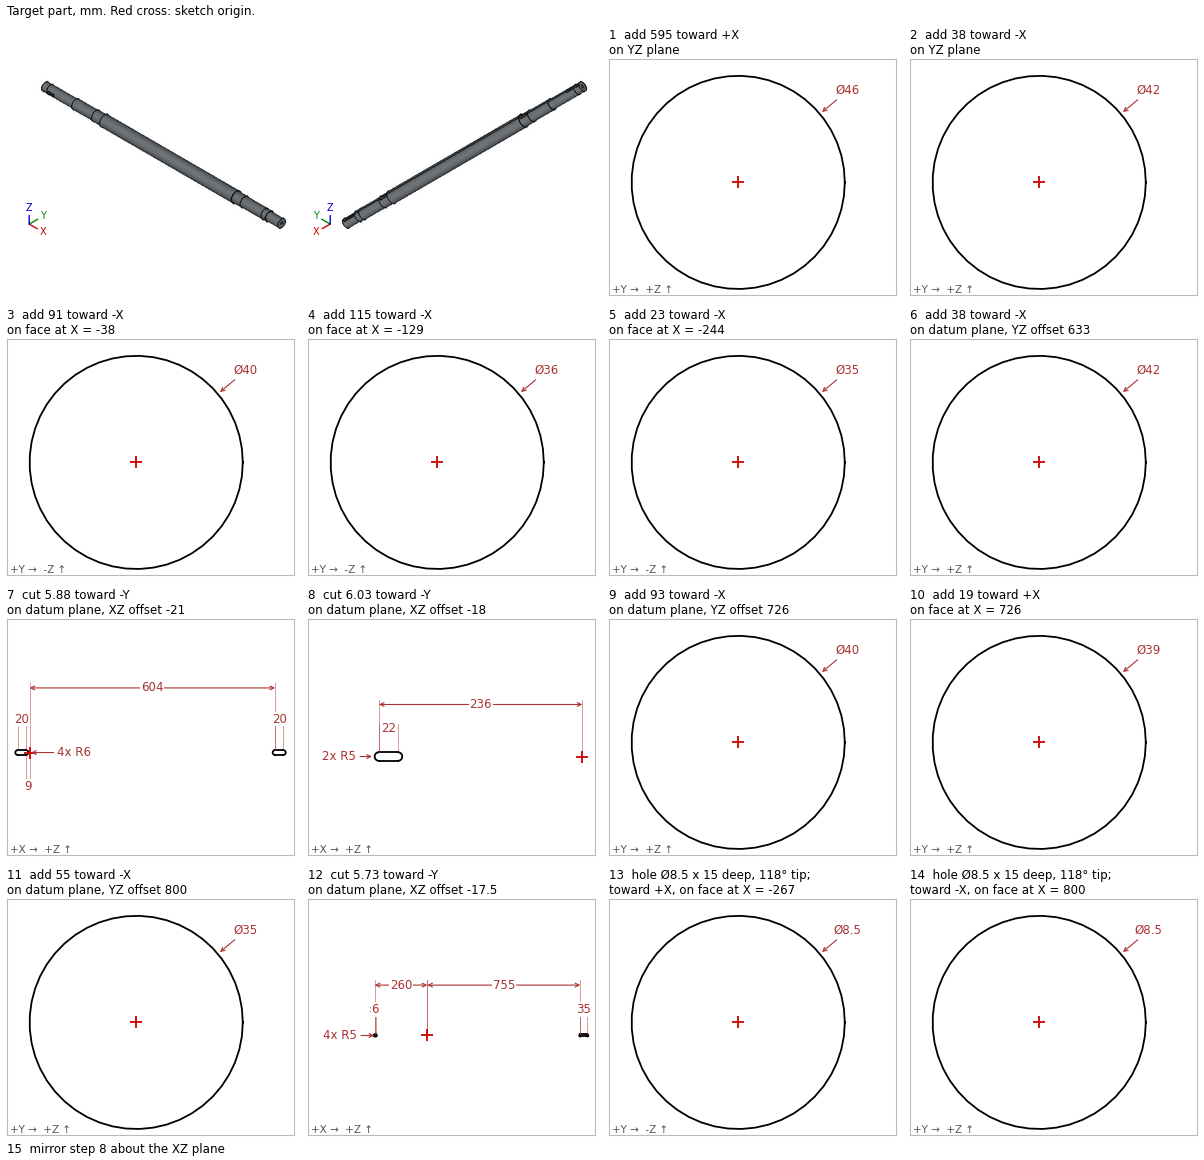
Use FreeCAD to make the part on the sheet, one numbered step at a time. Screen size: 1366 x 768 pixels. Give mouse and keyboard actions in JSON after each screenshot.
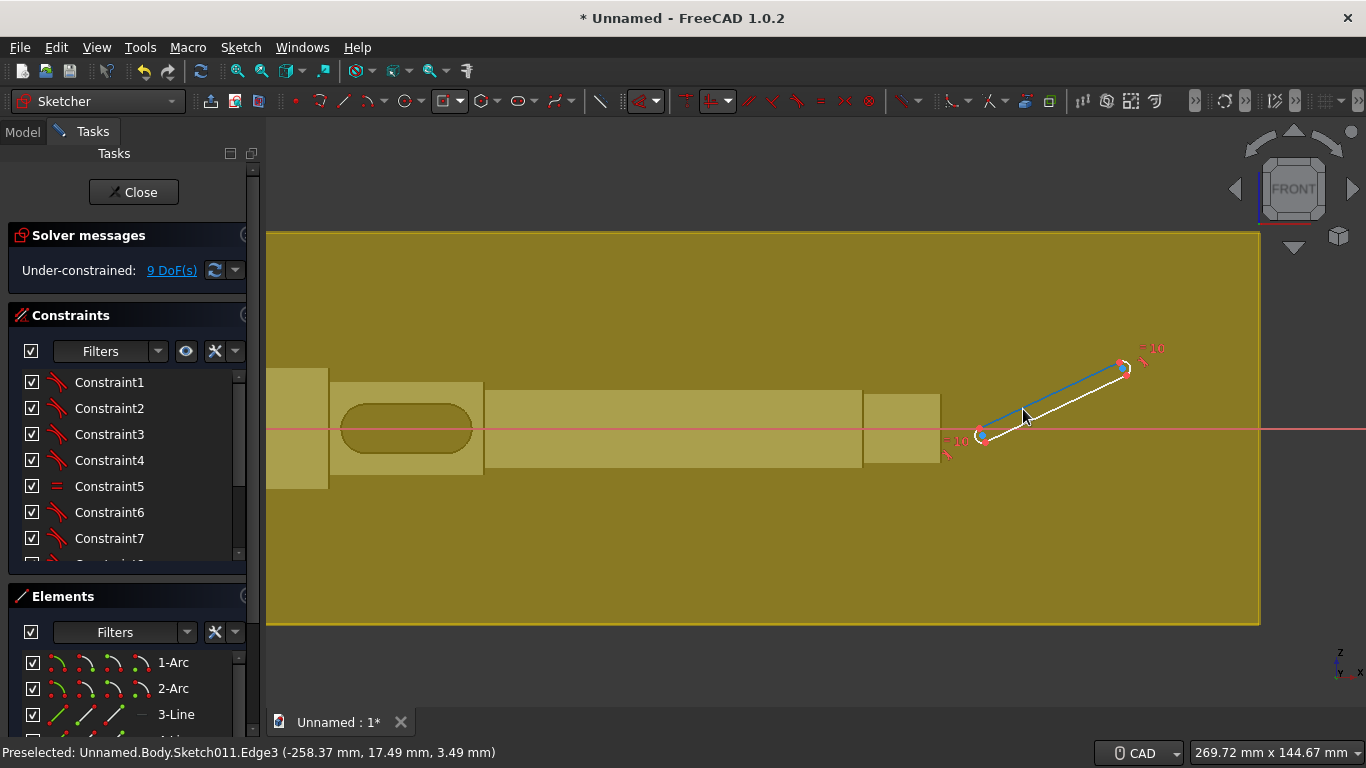
{"action": "left_click", "coordinate": [1021, 409]}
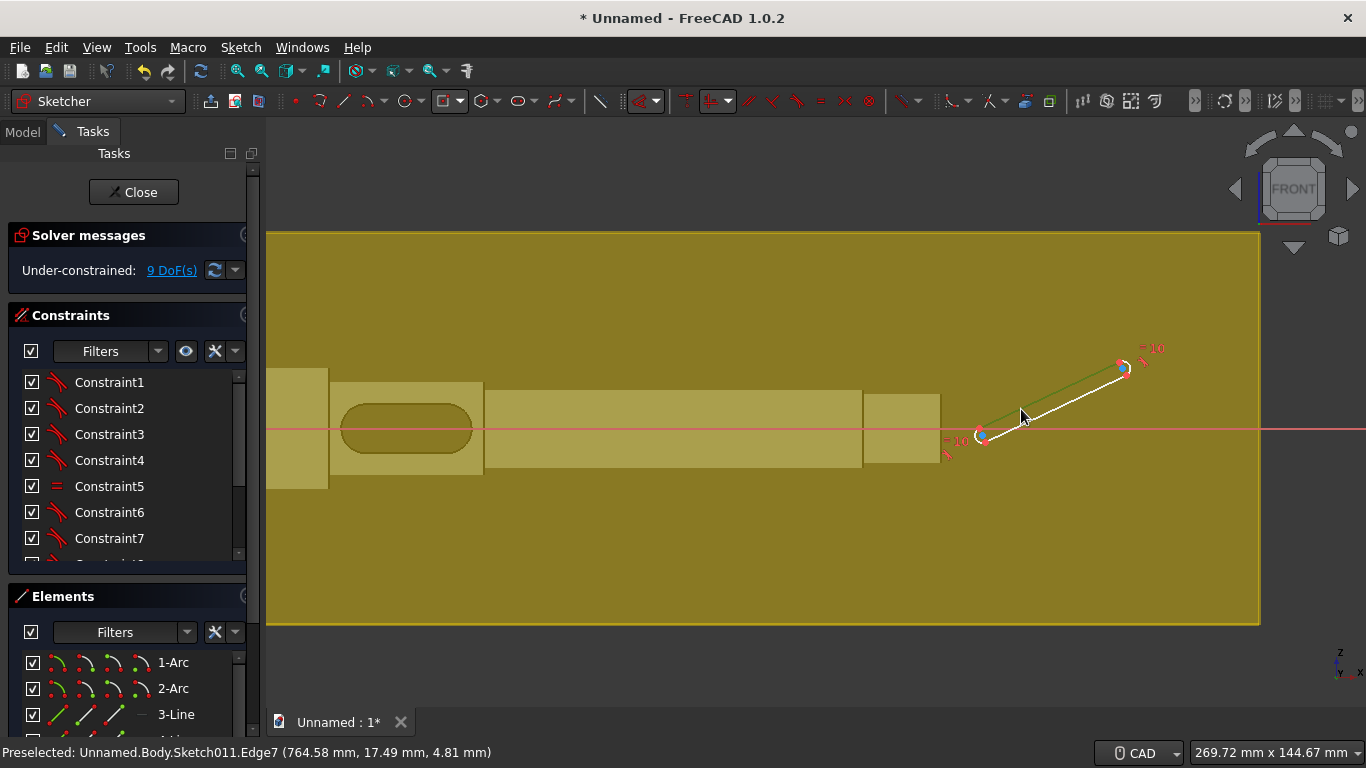
{"action": "key", "text": "h"}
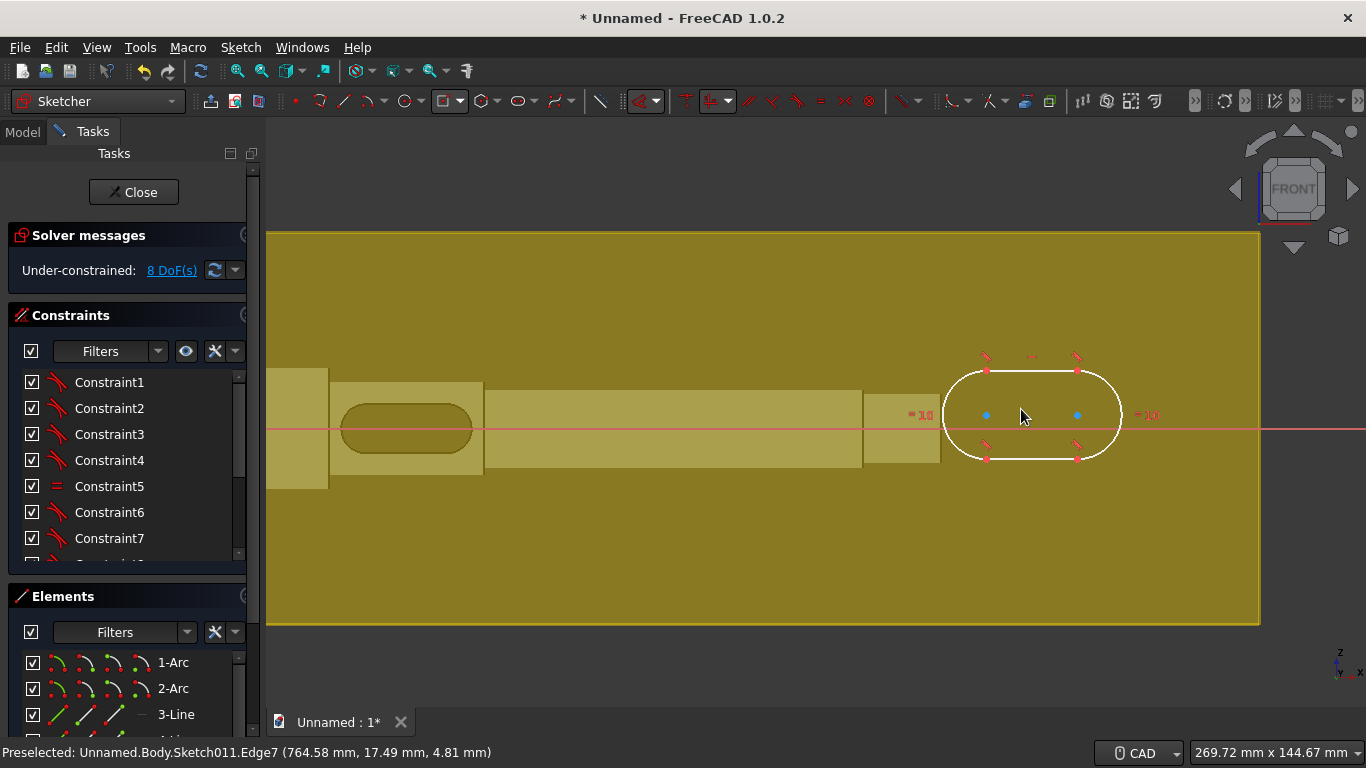
{"action": "scroll", "coordinate": [1024, 409], "scroll_direction": "down", "scroll_amount": 10}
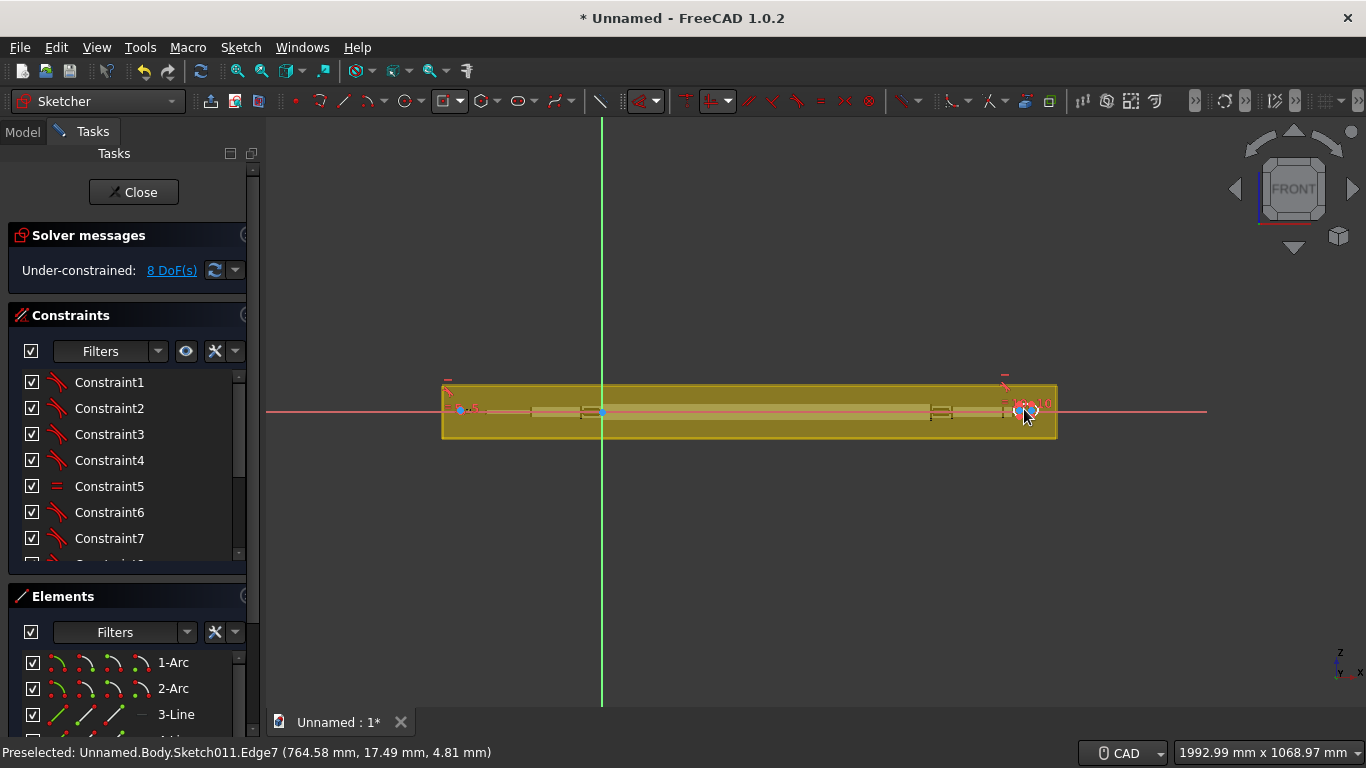
{"action": "scroll", "coordinate": [459, 411], "scroll_direction": "up", "scroll_amount": 13}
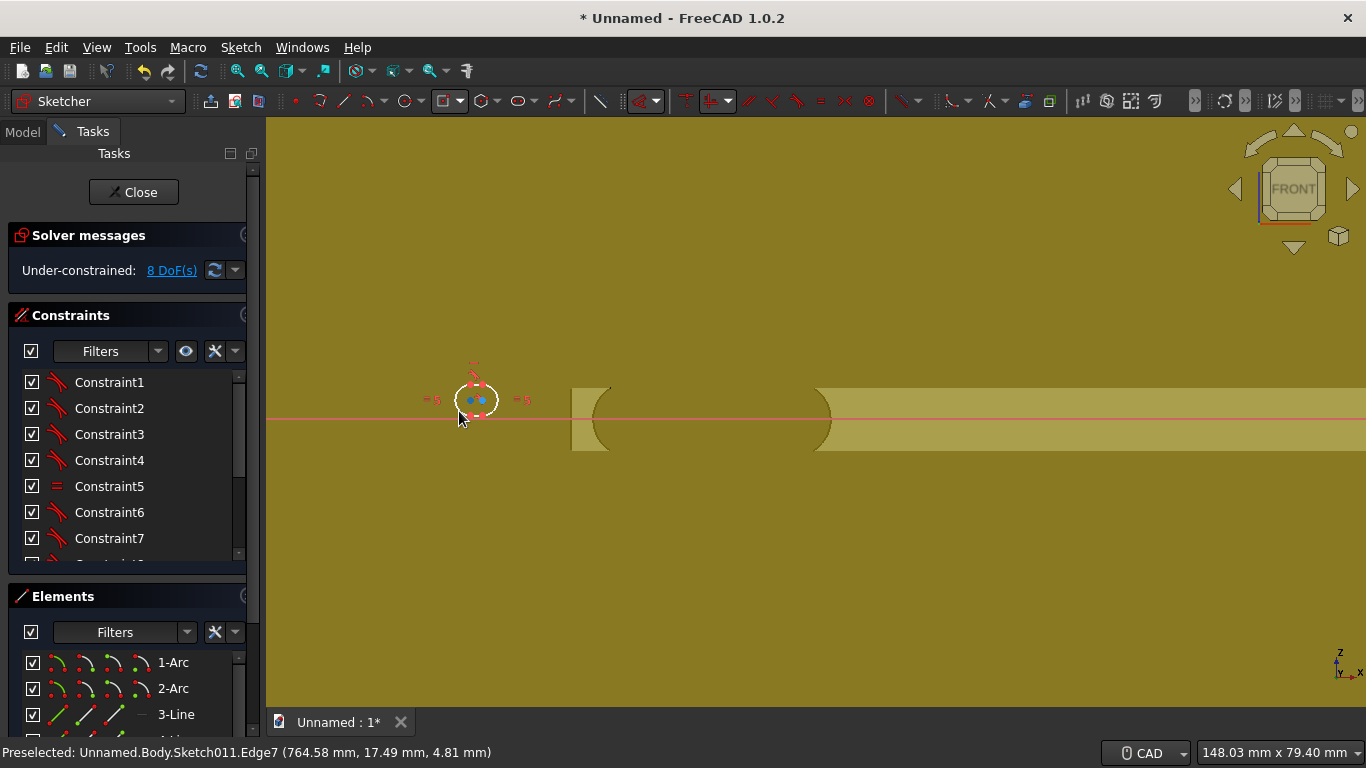
{"action": "left_click", "coordinate": [455, 400]}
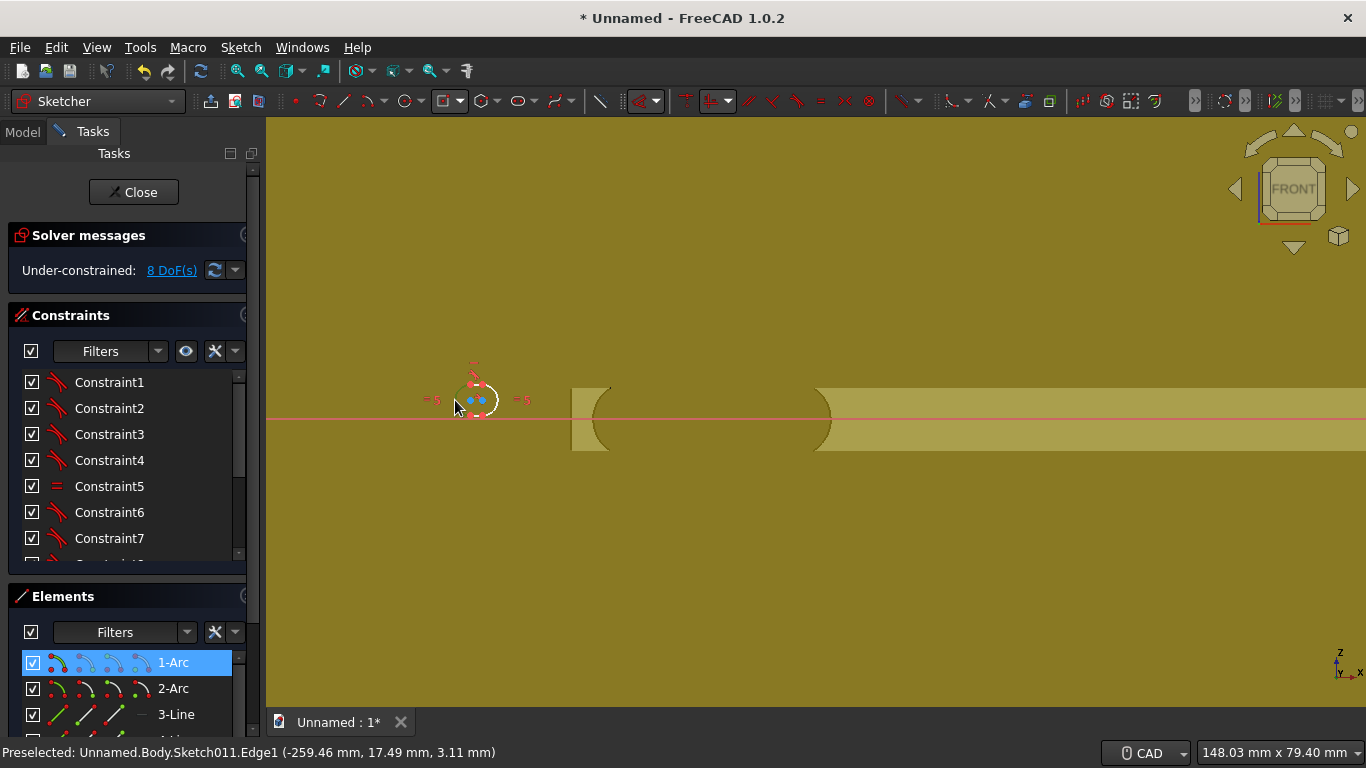
{"action": "scroll", "coordinate": [458, 411], "scroll_direction": "down", "scroll_amount": 13}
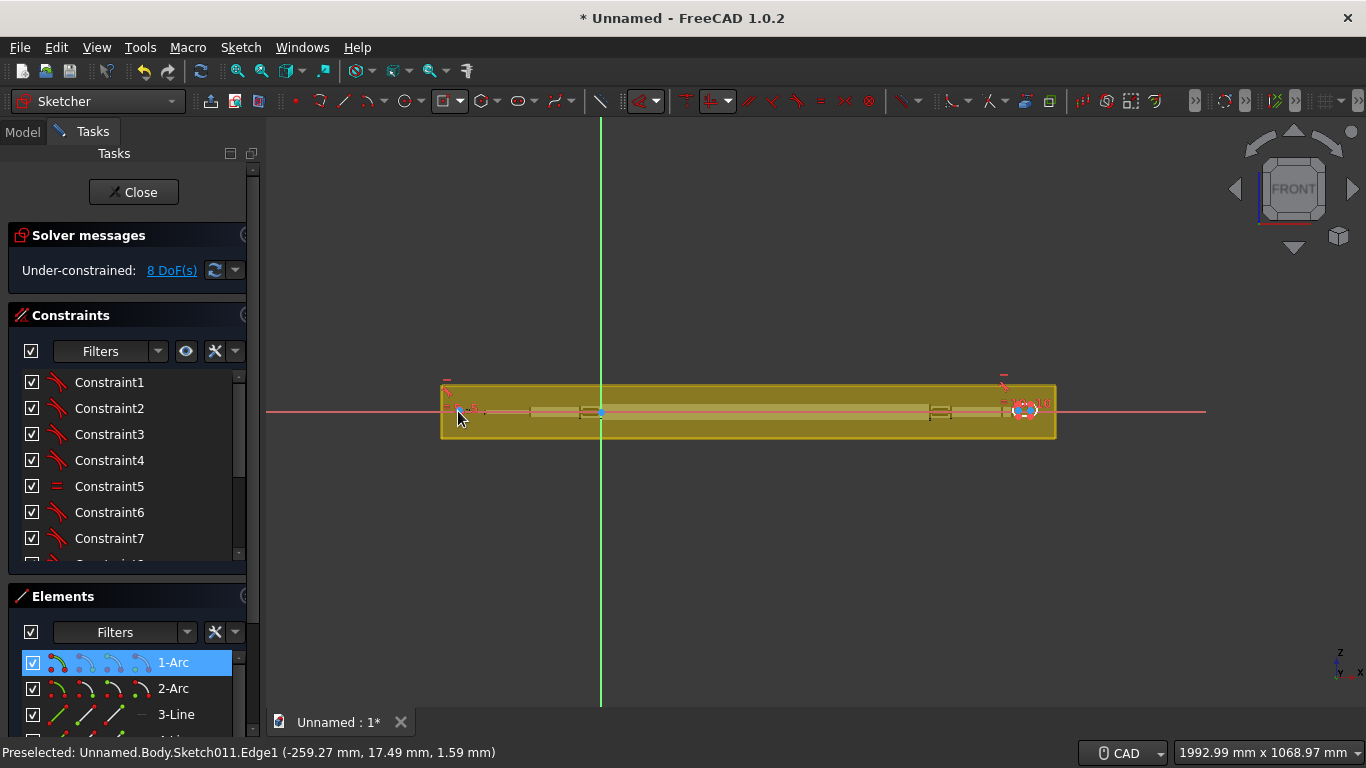
{"action": "scroll", "coordinate": [1014, 407], "scroll_direction": "up", "scroll_amount": 5}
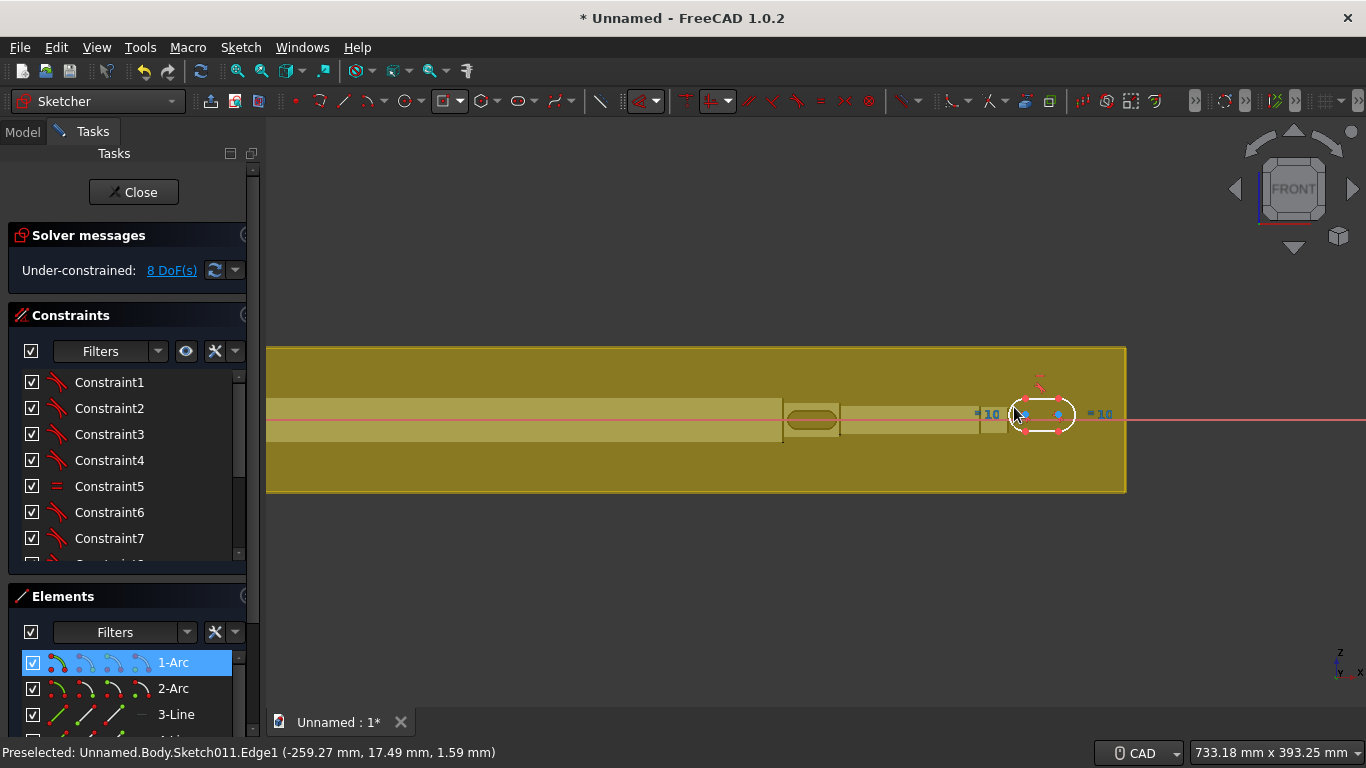
{"action": "left_click", "coordinate": [1012, 405]}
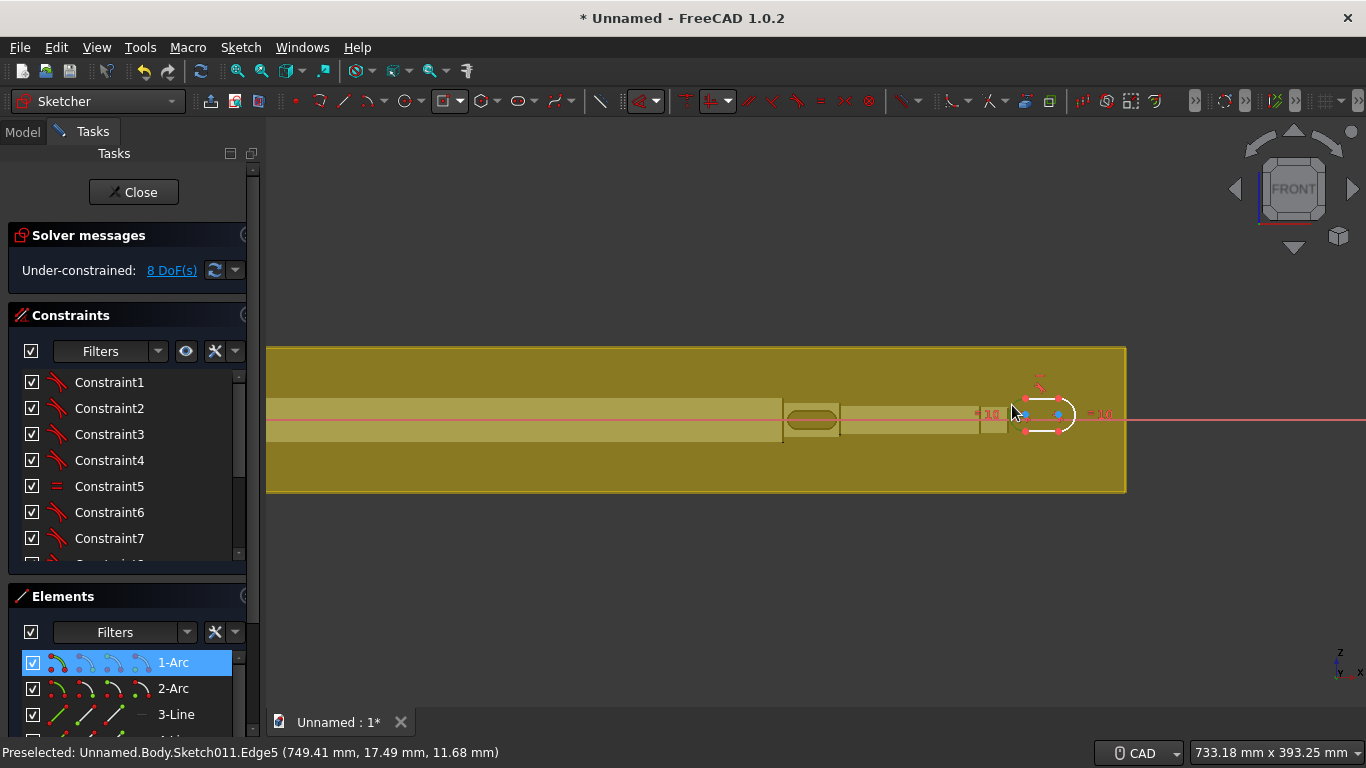
{"action": "key", "text": "e"}